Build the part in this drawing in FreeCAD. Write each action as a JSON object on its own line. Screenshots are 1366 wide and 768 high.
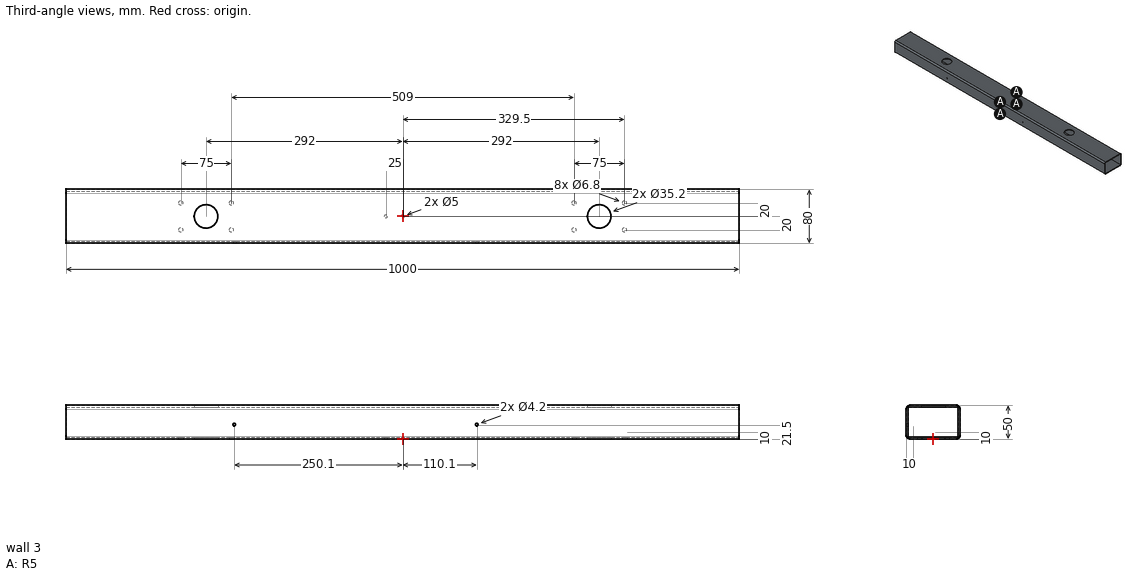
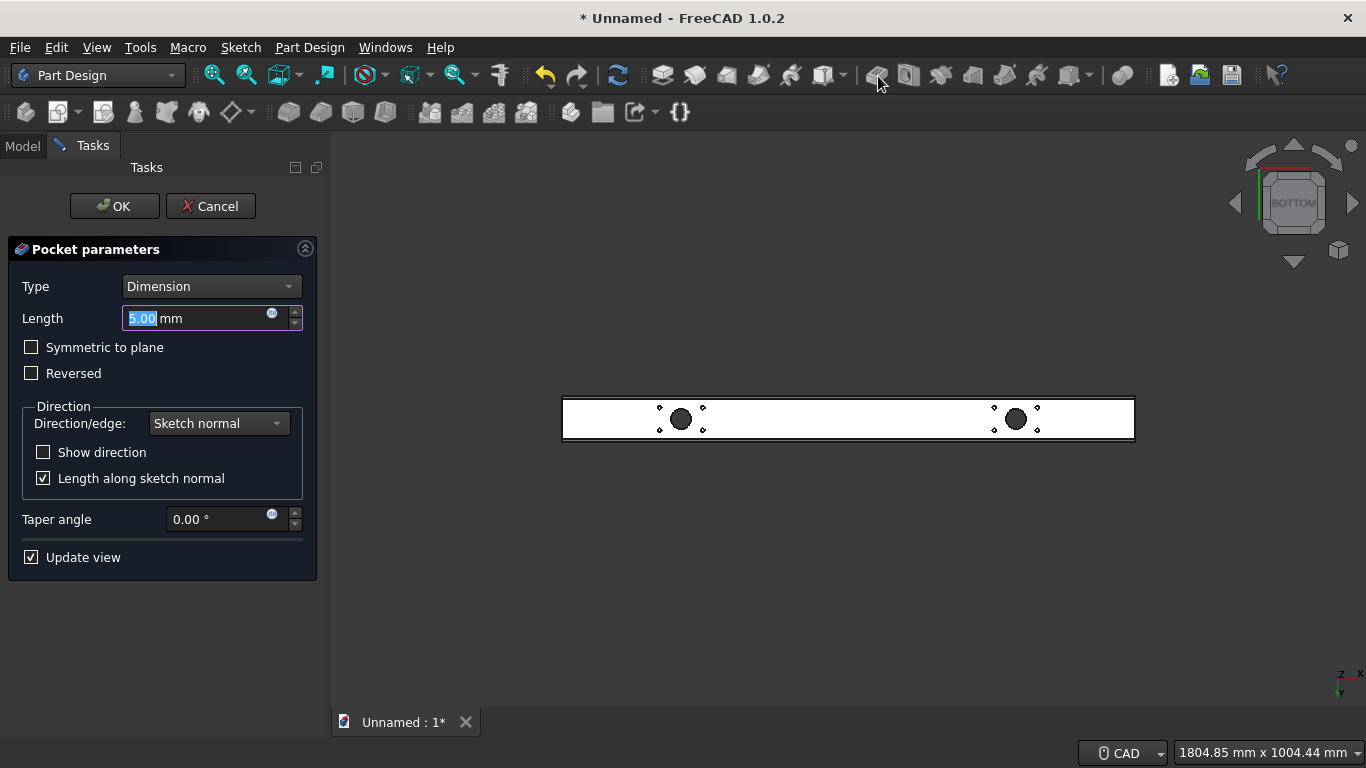
{"action": "type", "text": "10"}
{"action": "key", "text": "Tab"}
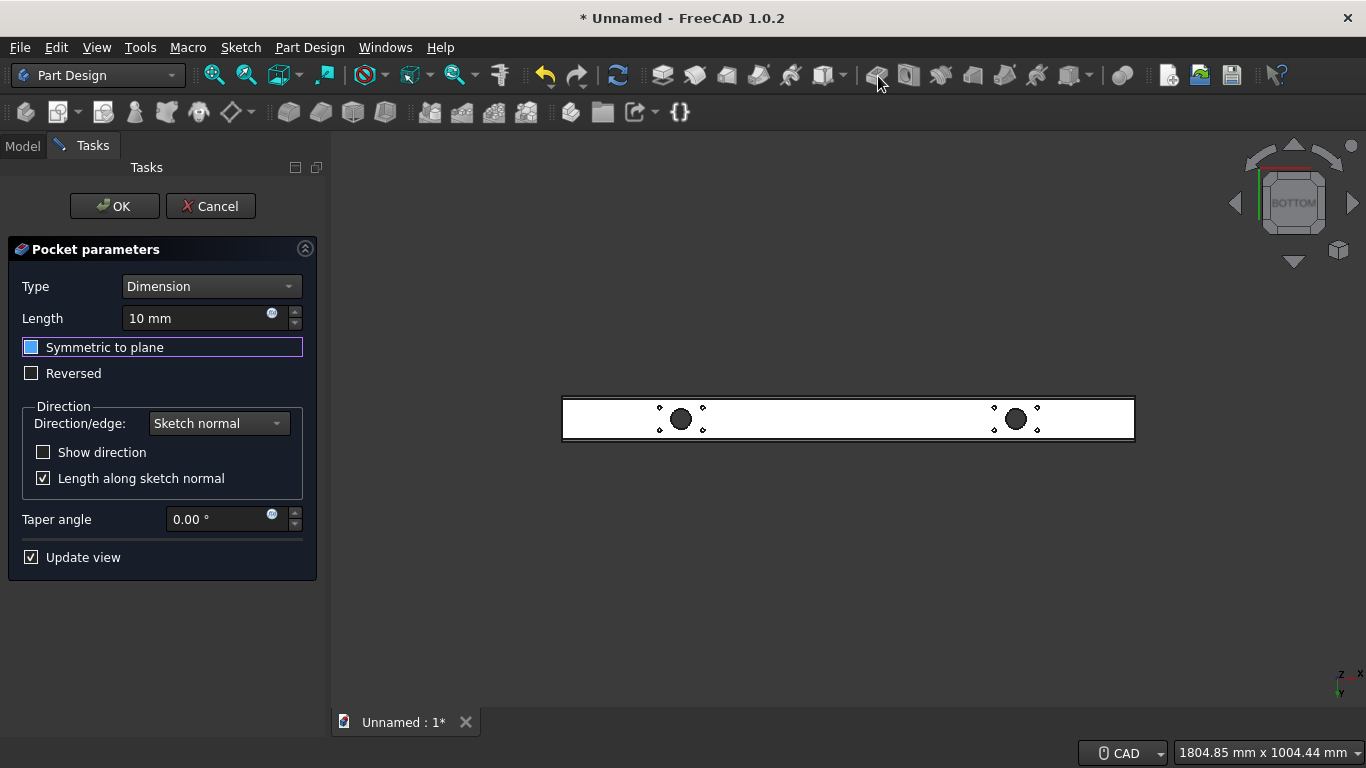
{"action": "left_click", "coordinate": [30, 373]}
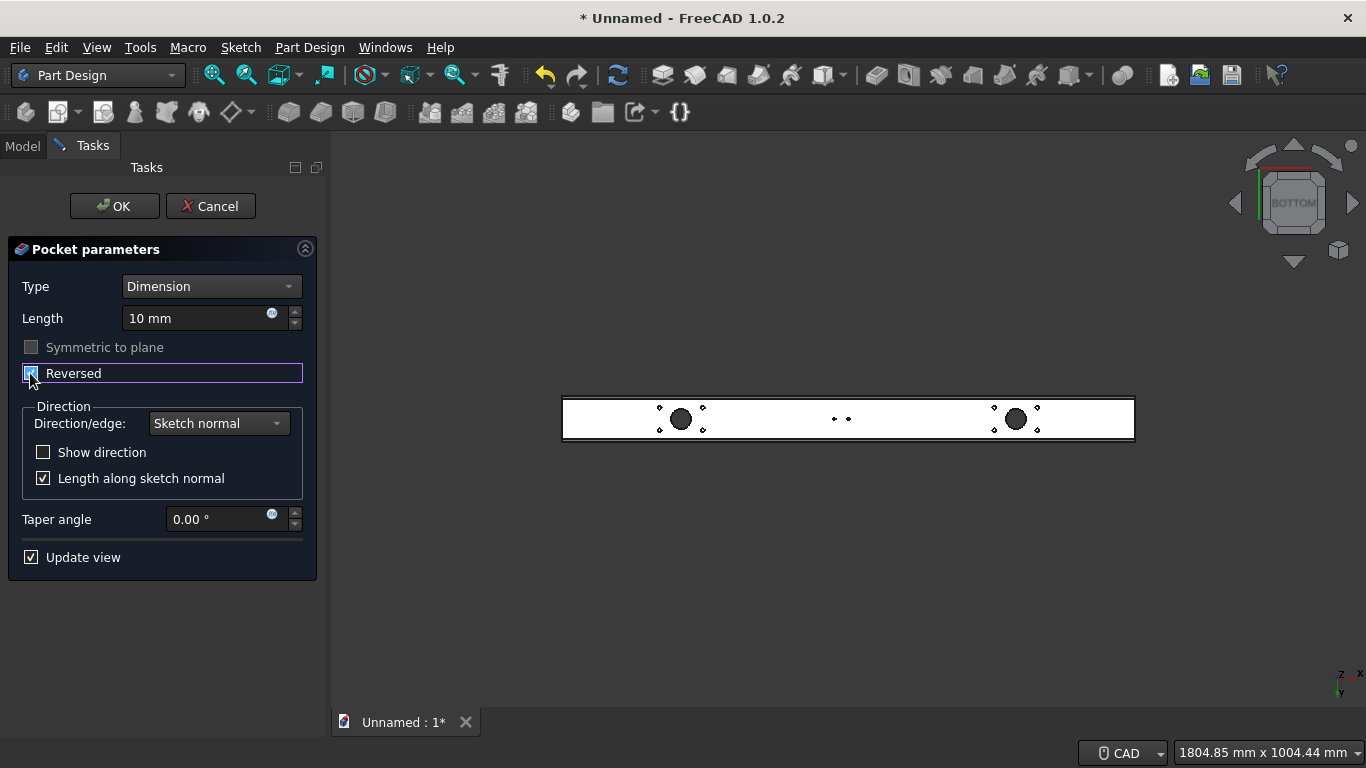
{"action": "left_click", "coordinate": [115, 206]}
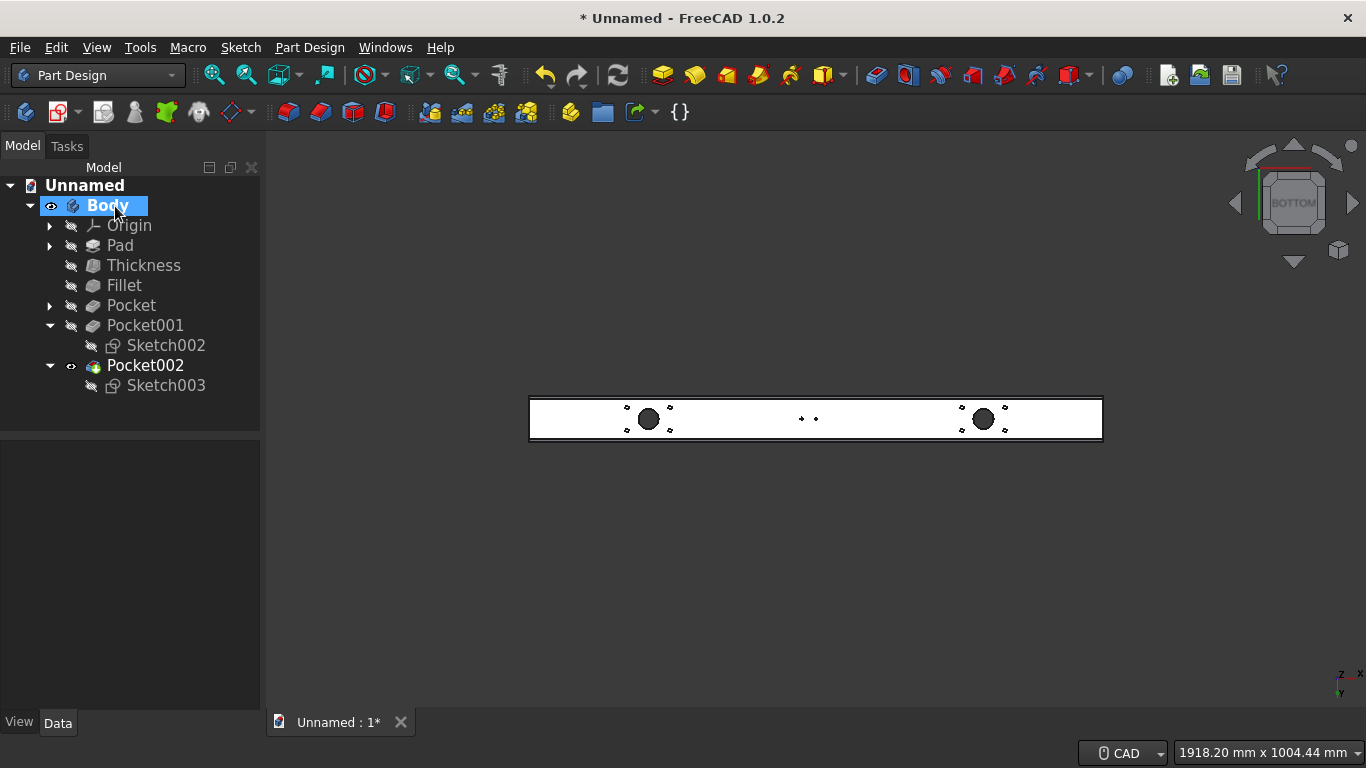
{"action": "key", "text": "0"}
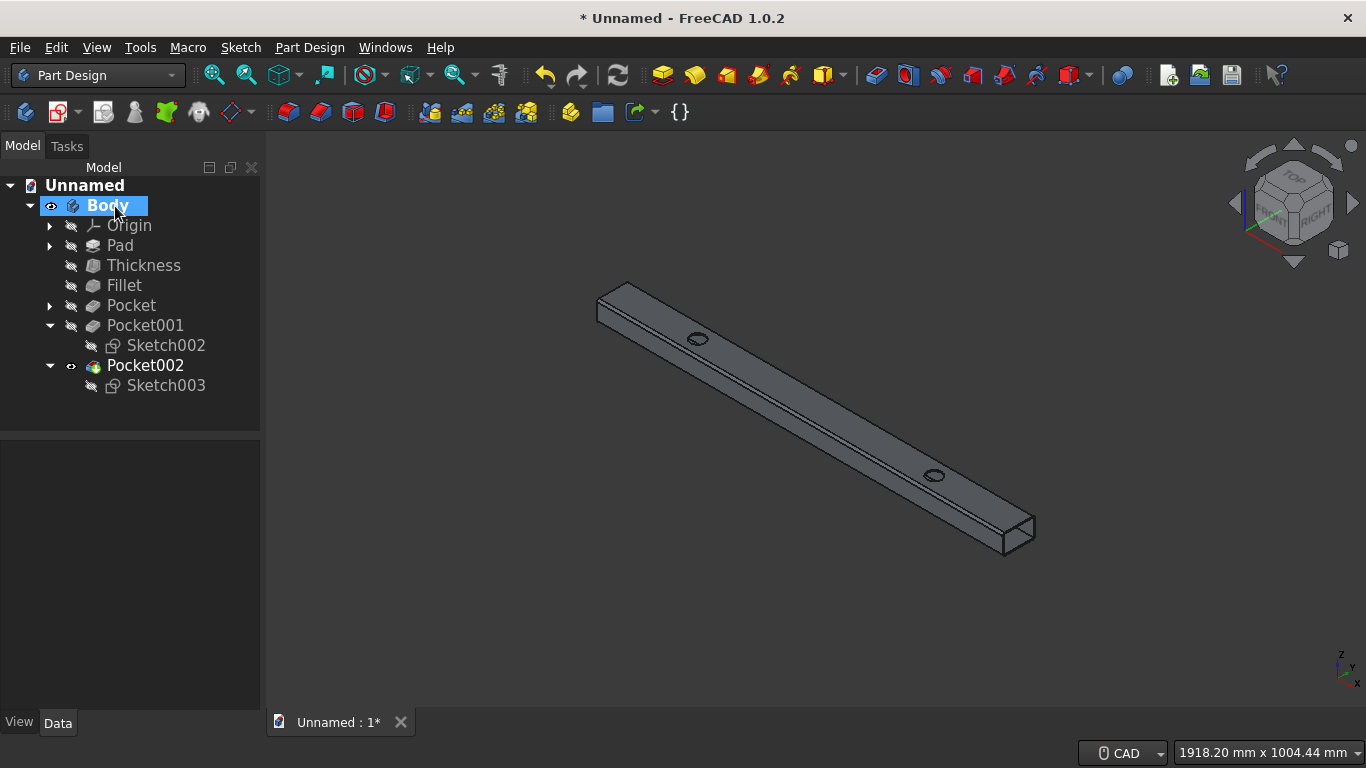
{"action": "key", "text": "1"}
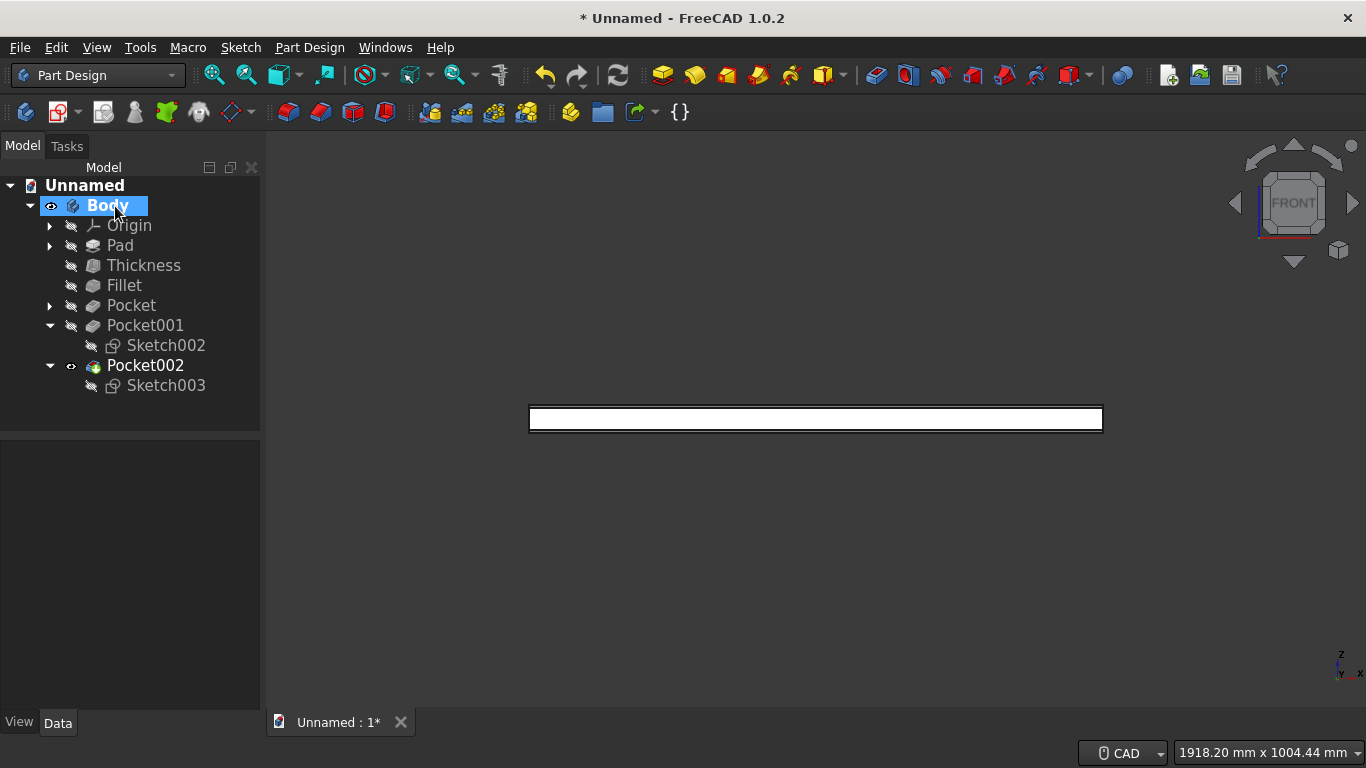
{"action": "left_click", "coordinate": [1062, 418]}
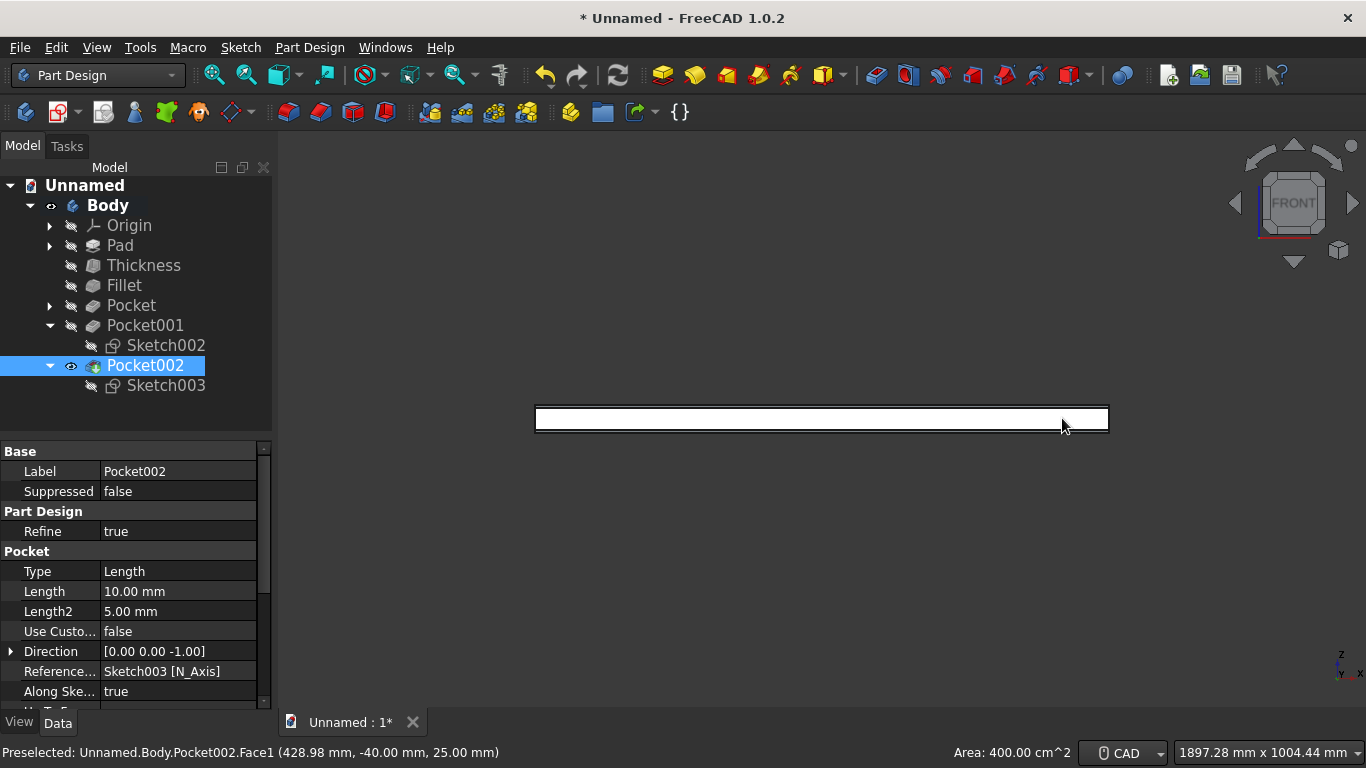
{"action": "left_click", "coordinate": [58, 112]}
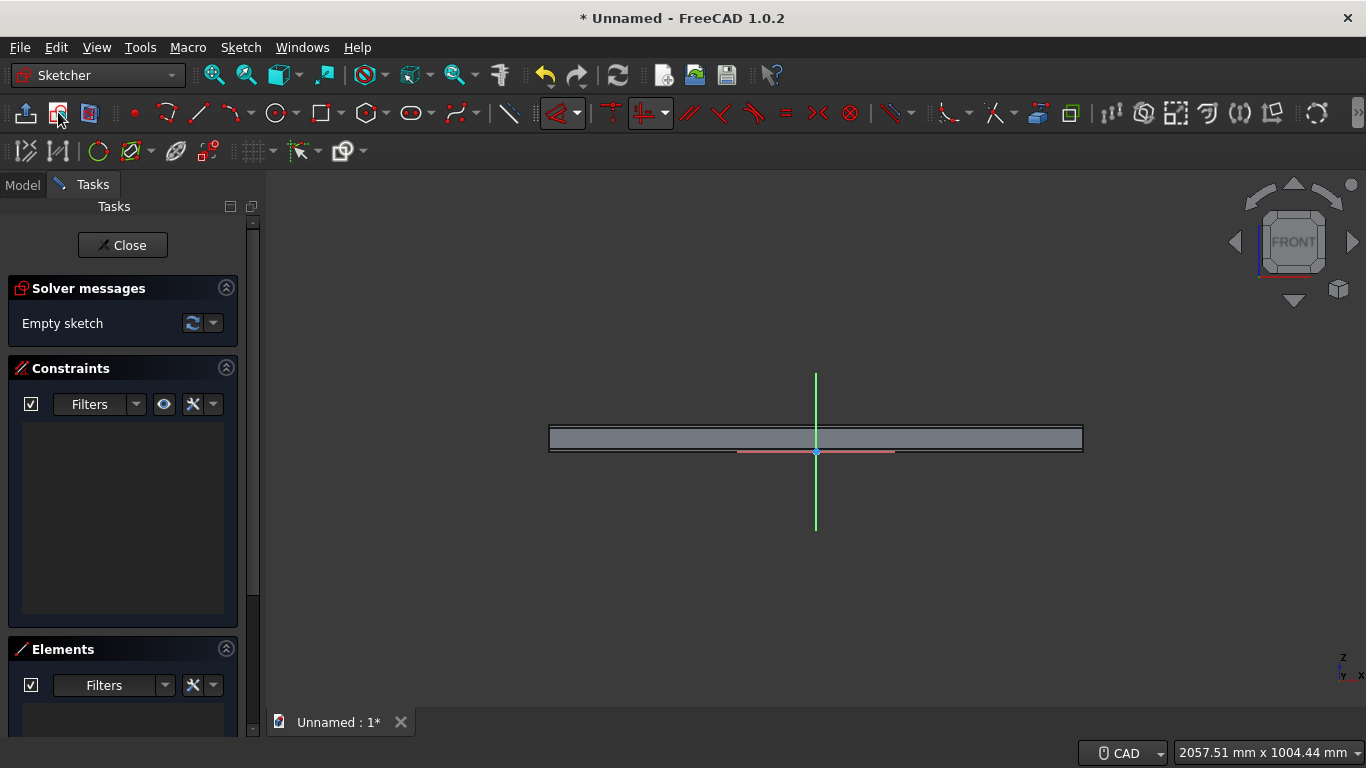
{"action": "scroll", "coordinate": [792, 449], "scroll_direction": "up", "scroll_amount": 6}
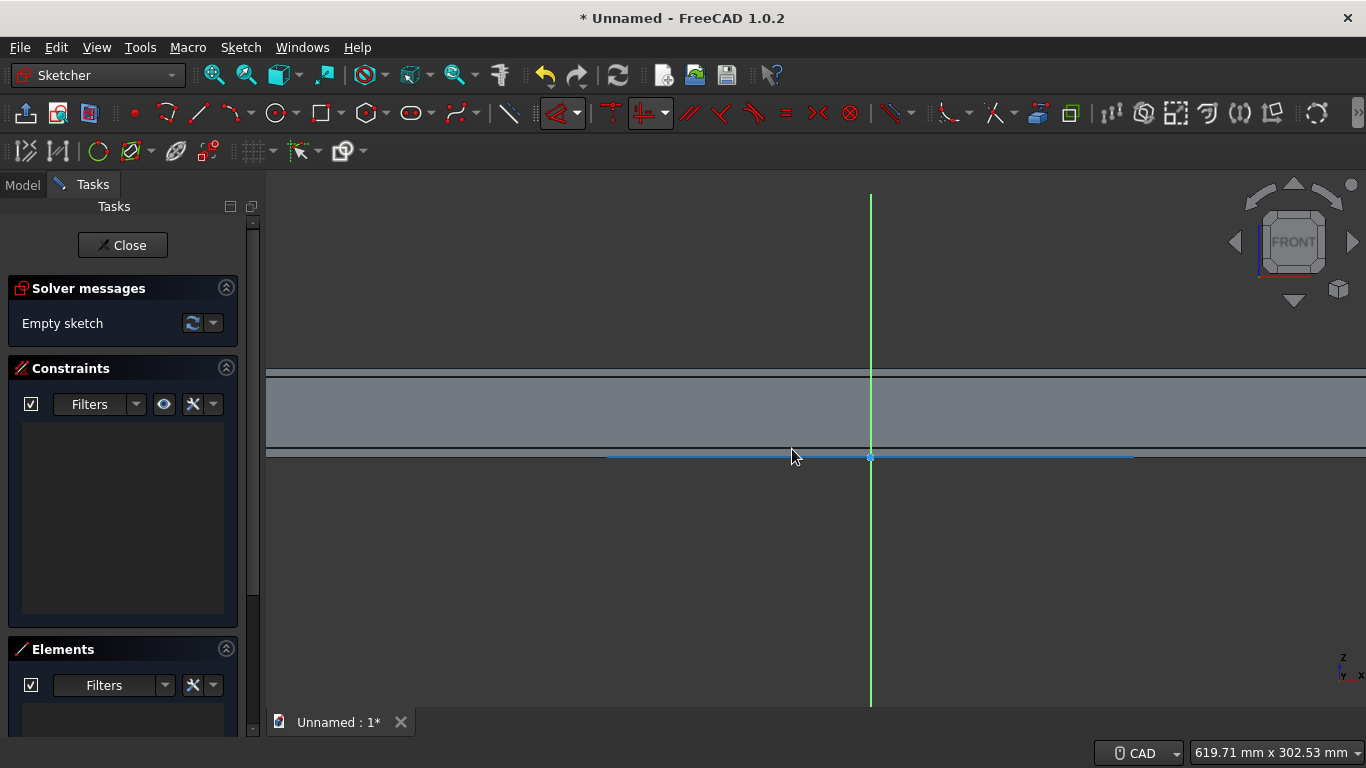
{"action": "left_click", "coordinate": [276, 114]}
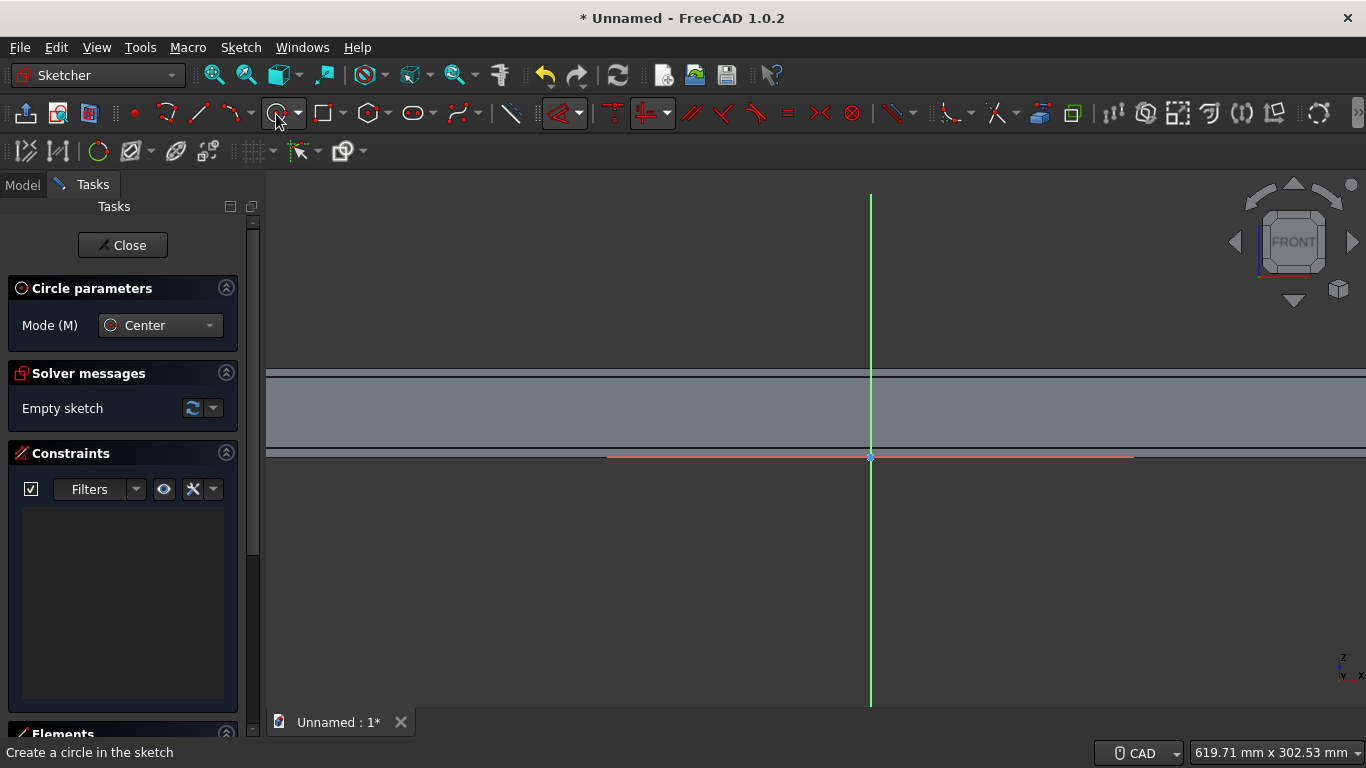
{"action": "scroll", "coordinate": [1066, 419], "scroll_direction": "up", "scroll_amount": 10}